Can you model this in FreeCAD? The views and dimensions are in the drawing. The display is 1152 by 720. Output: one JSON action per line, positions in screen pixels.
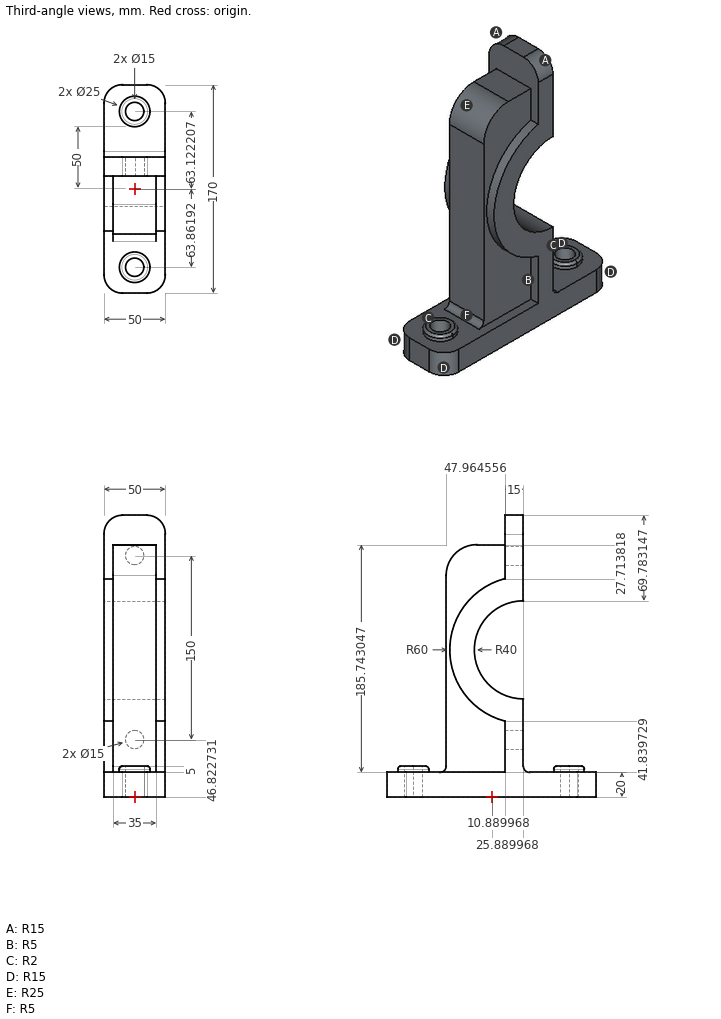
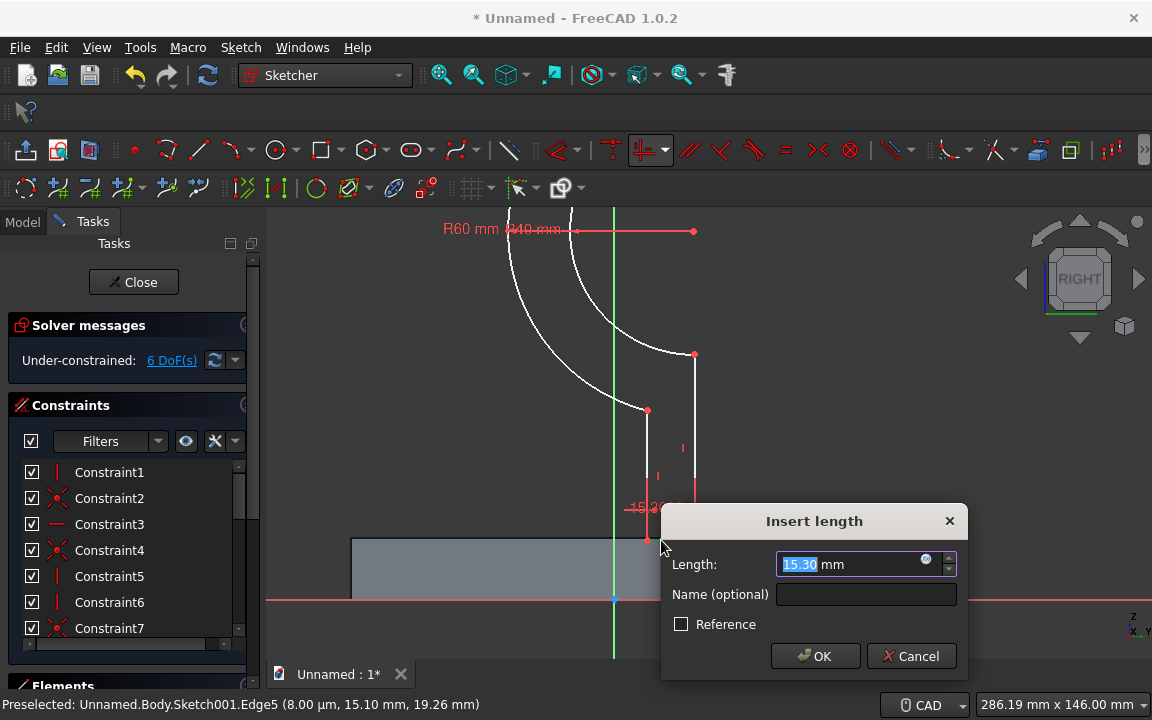
{"action": "type", "text": "15"}
{"action": "key", "text": "Return"}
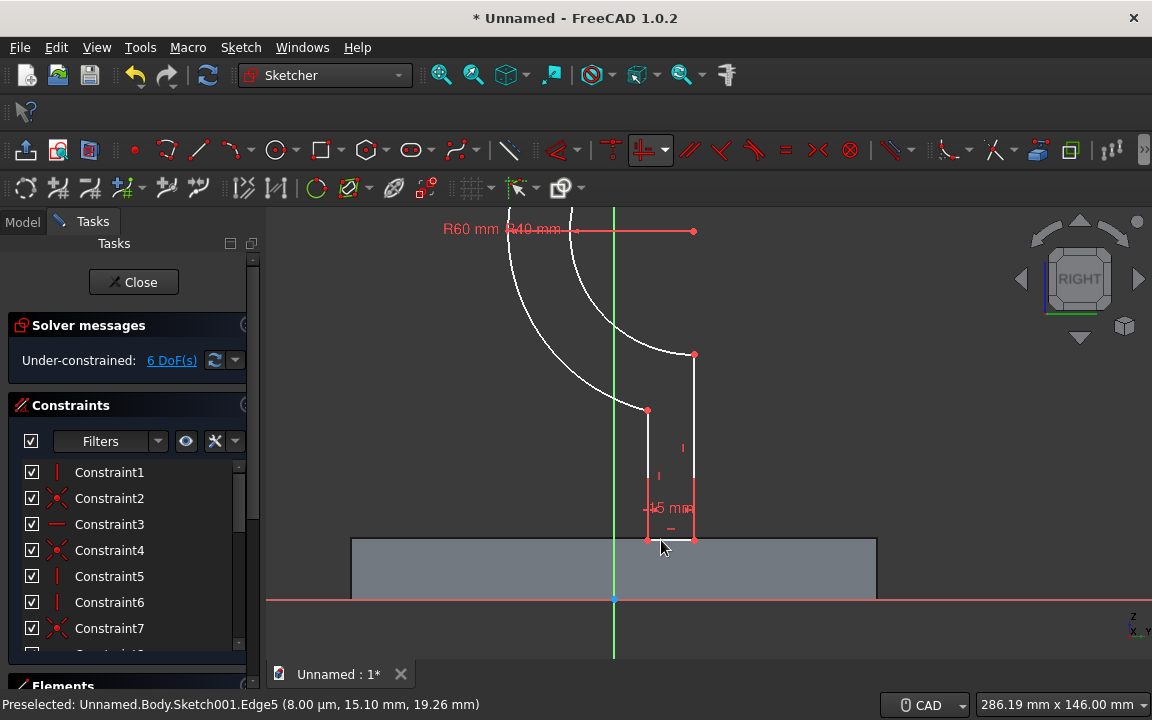
{"action": "left_click", "coordinate": [648, 540]}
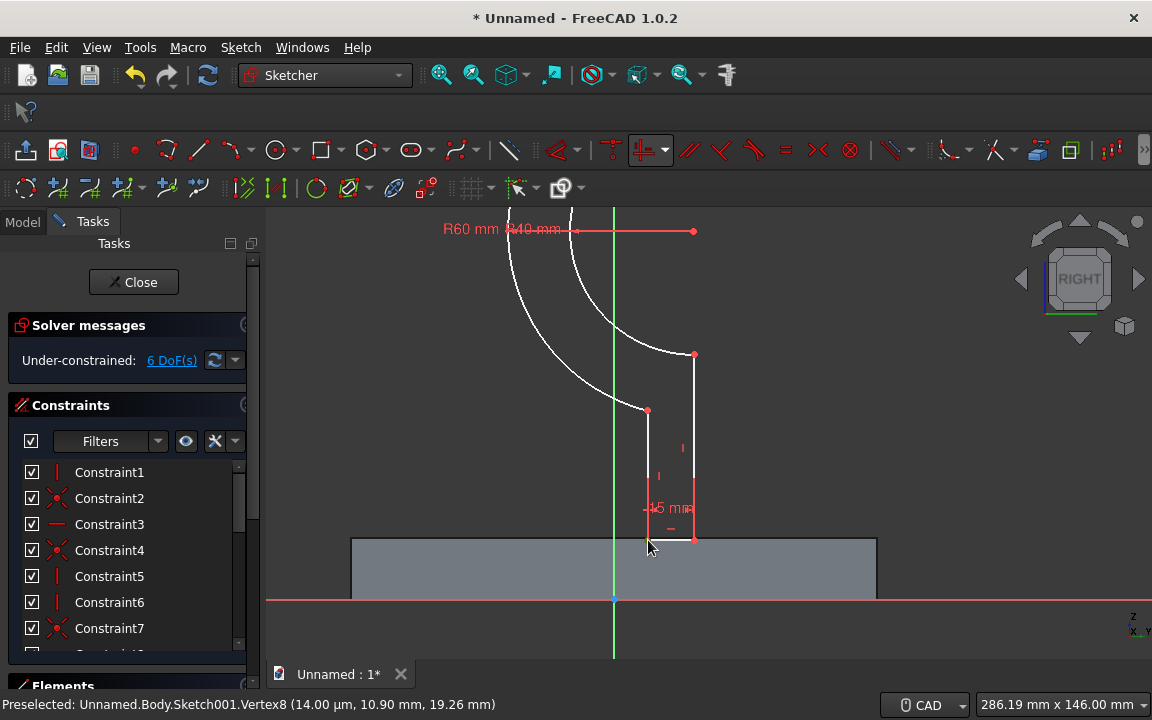
{"action": "key", "text": "i"}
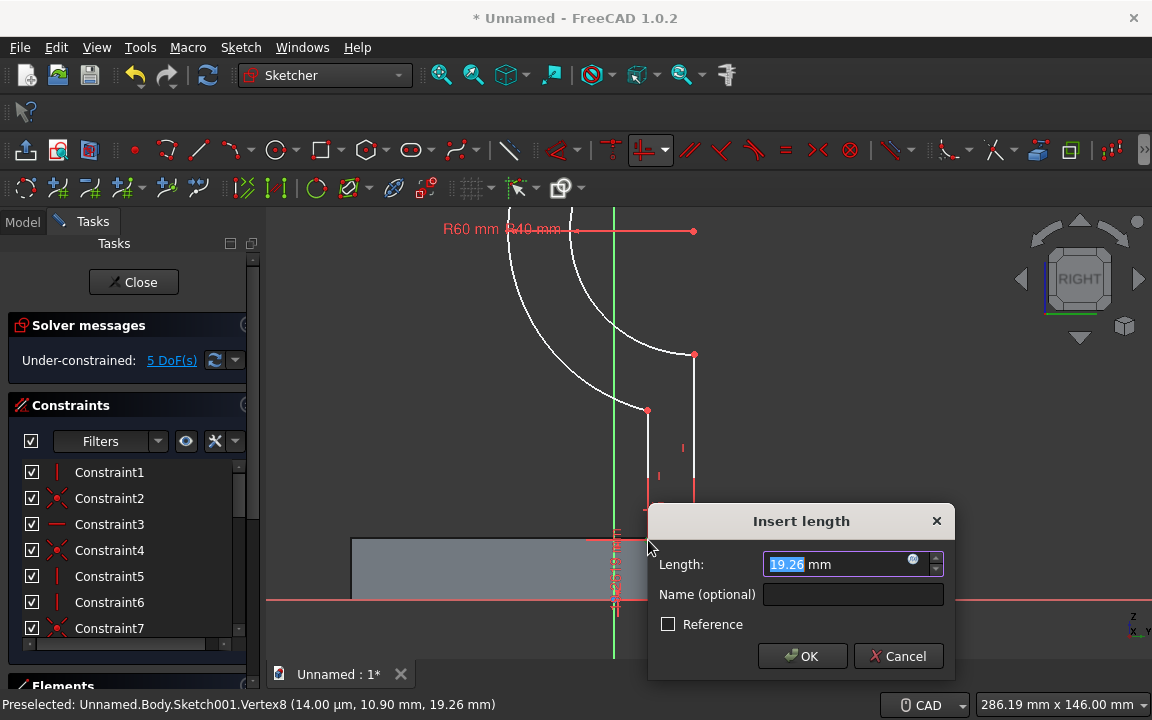
{"action": "type", "text": "20"}
{"action": "key", "text": "Return"}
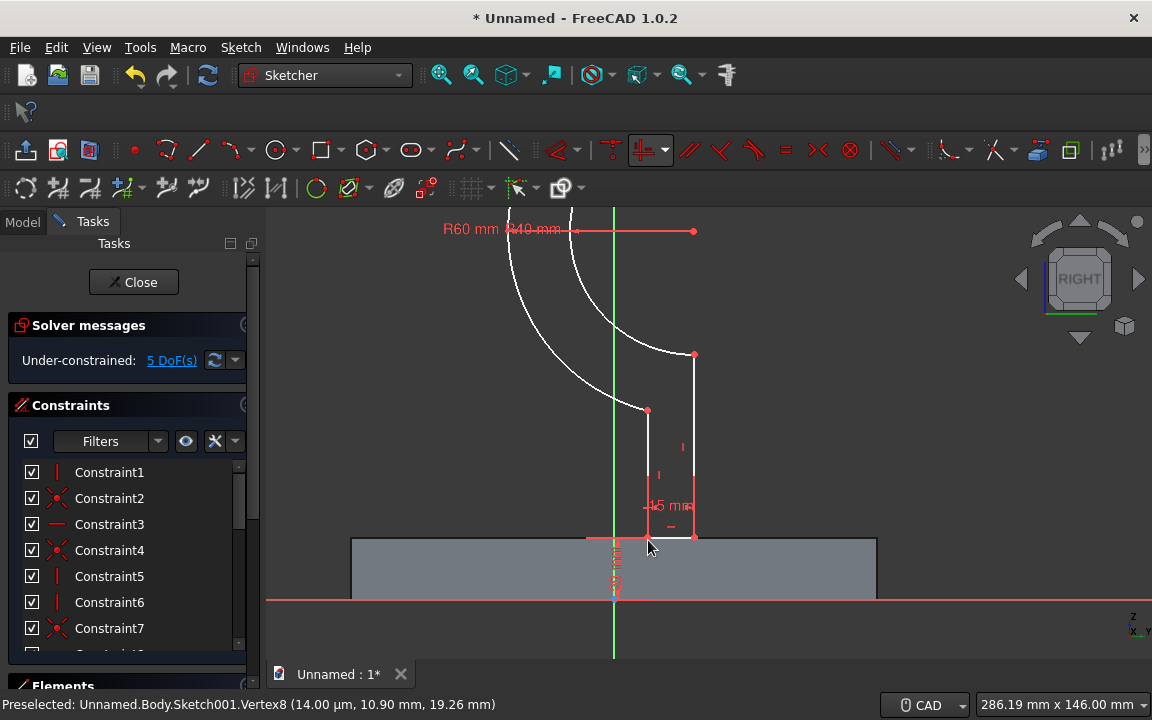
{"action": "scroll", "coordinate": [663, 543], "scroll_direction": "down", "scroll_amount": 5}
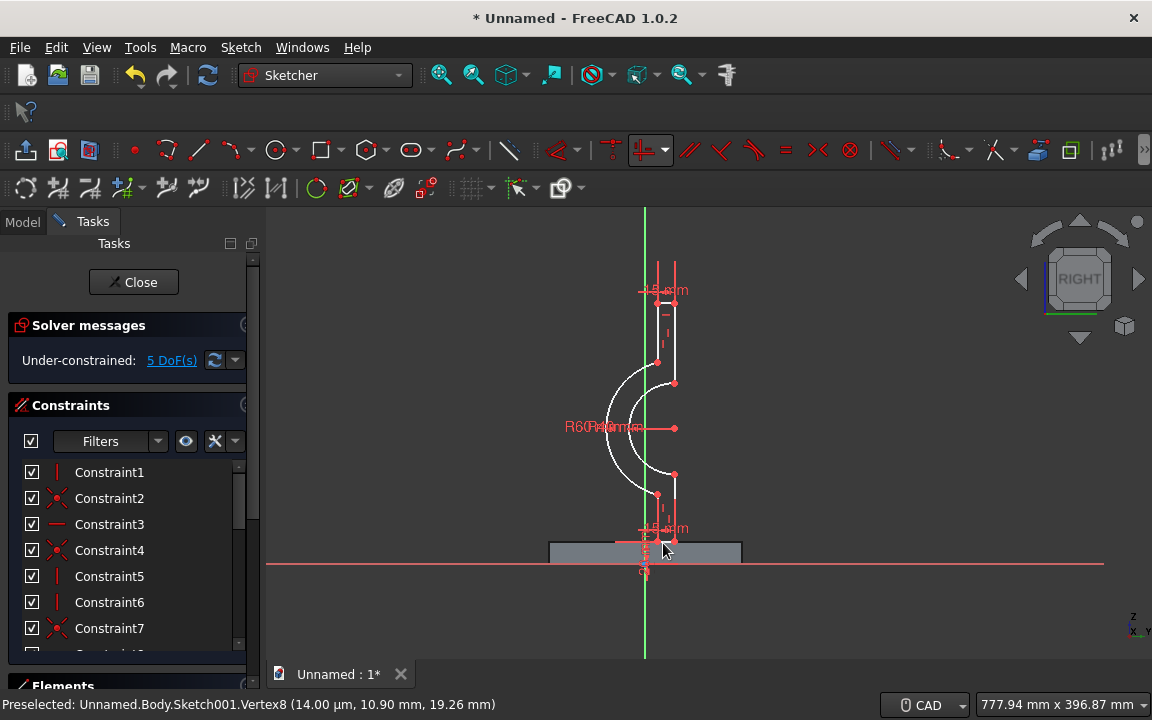
{"action": "left_click", "coordinate": [675, 359]}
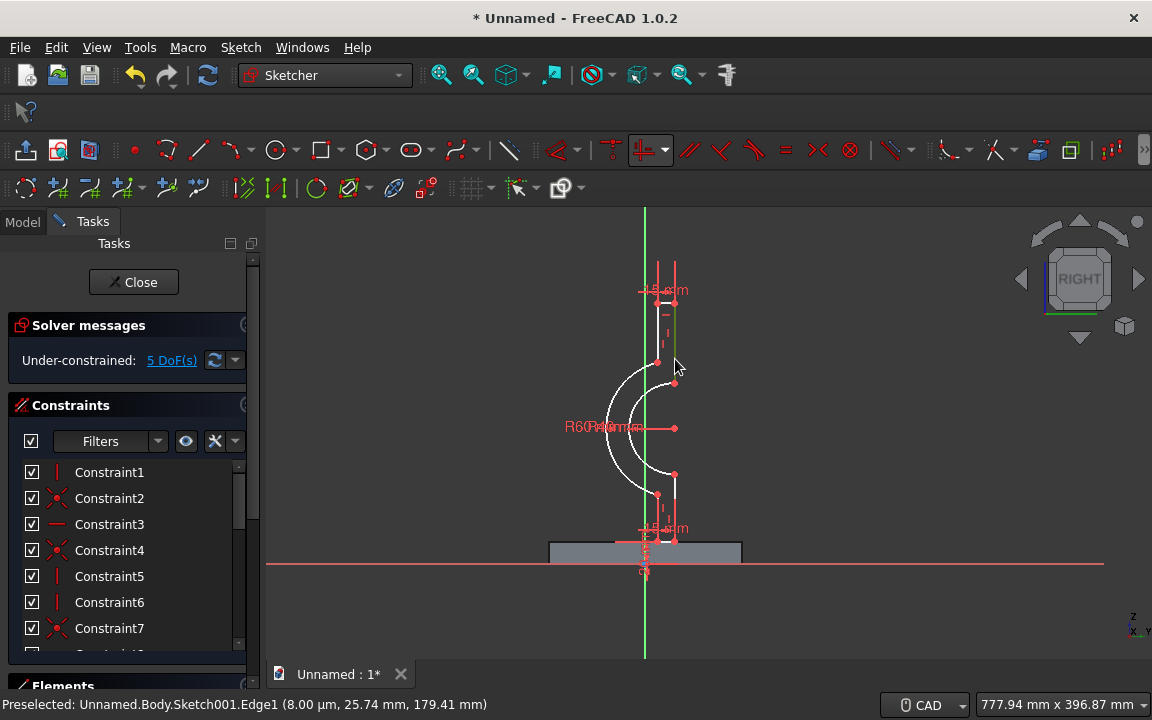
{"action": "key", "text": "i"}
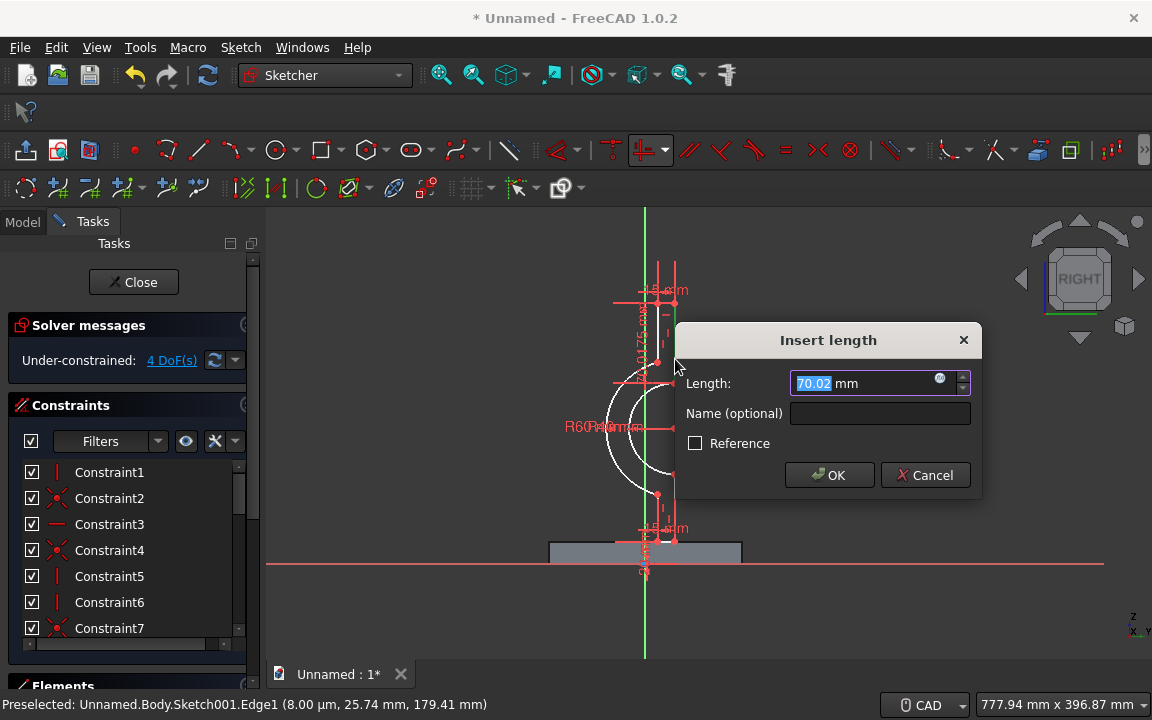
{"action": "type", "text": "69.783147"}
{"action": "key", "text": "Return"}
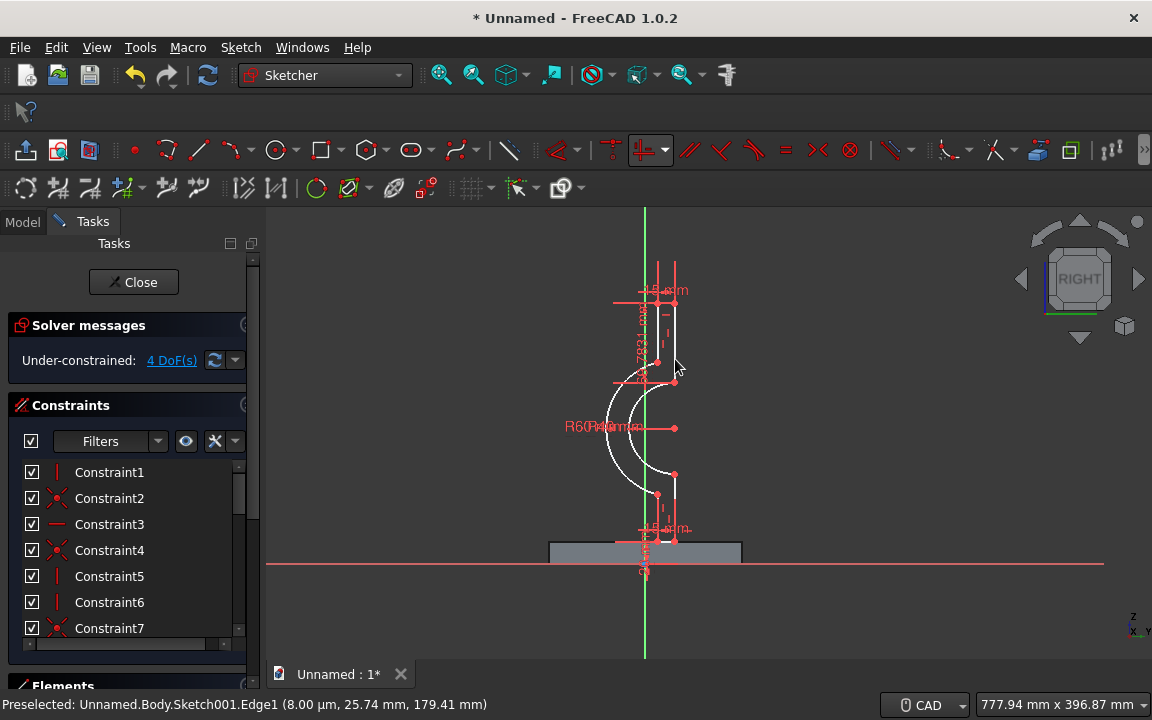
{"action": "left_click", "coordinate": [658, 513]}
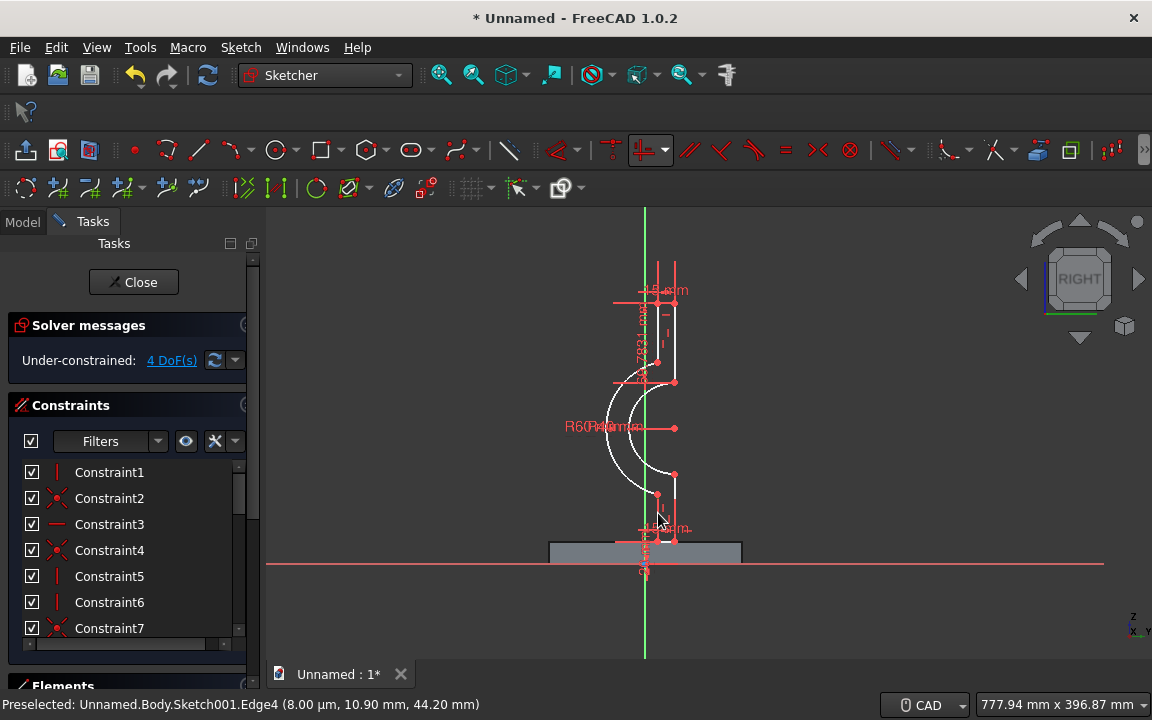
{"action": "left_click", "coordinate": [580, 150]}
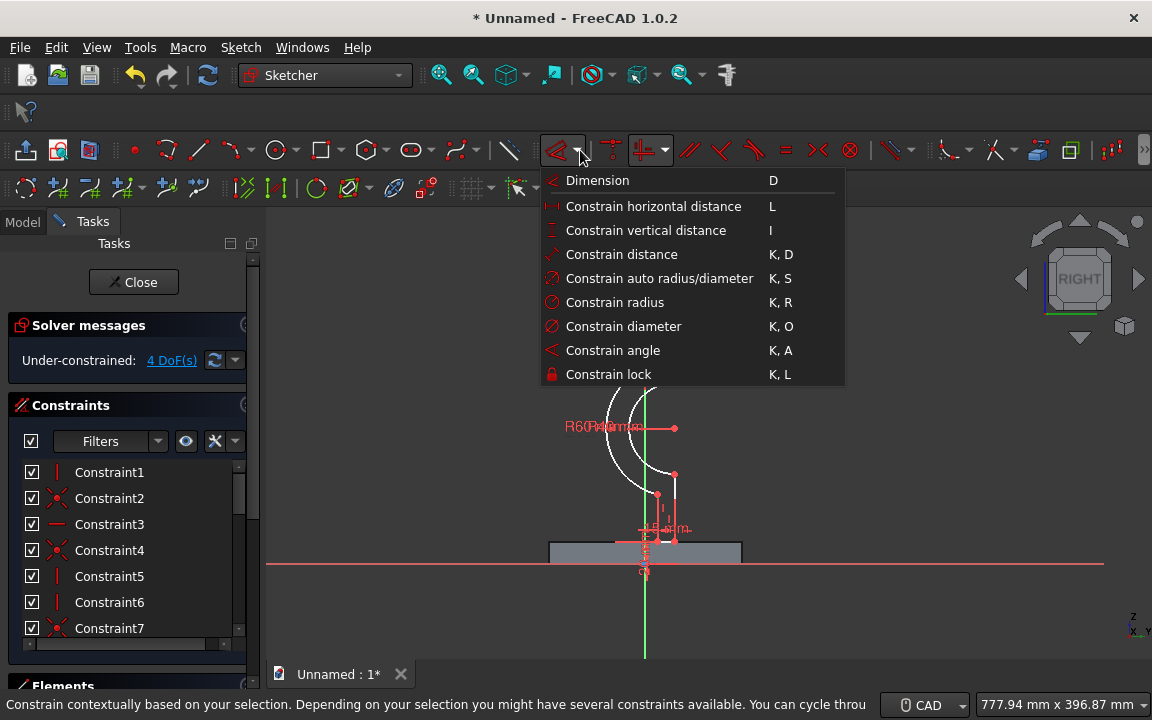
{"action": "left_click", "coordinate": [693, 230]}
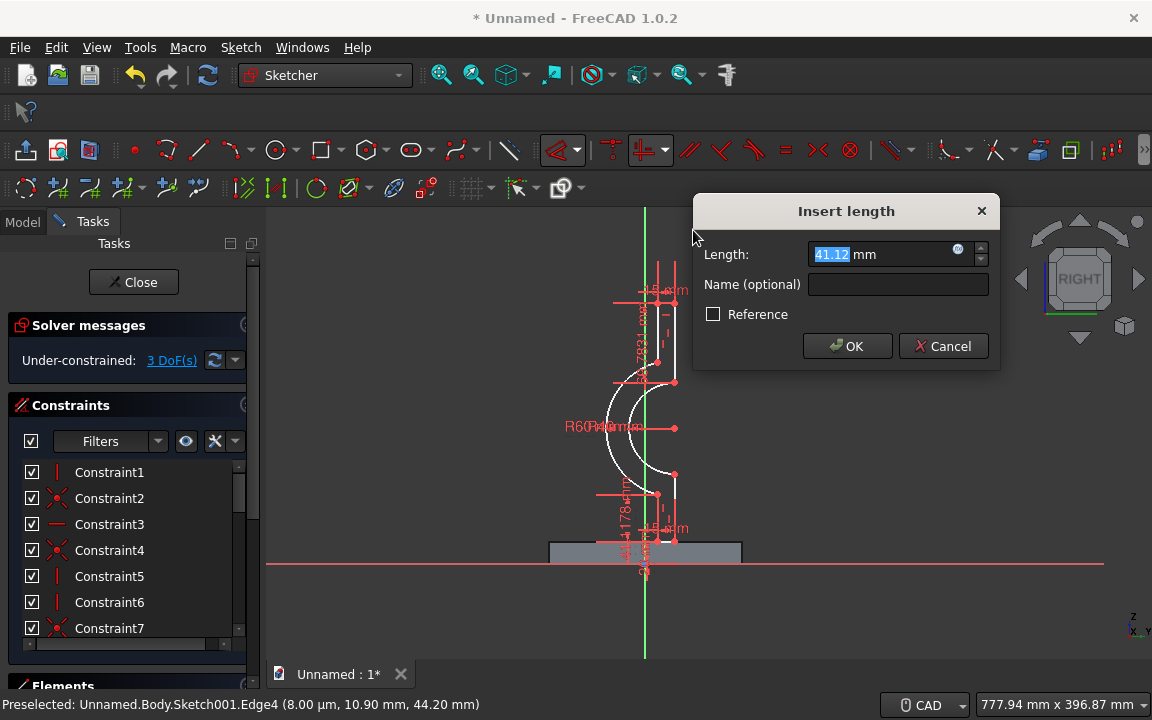
{"action": "type", "text": "41.839729"}
{"action": "key", "text": "Return"}